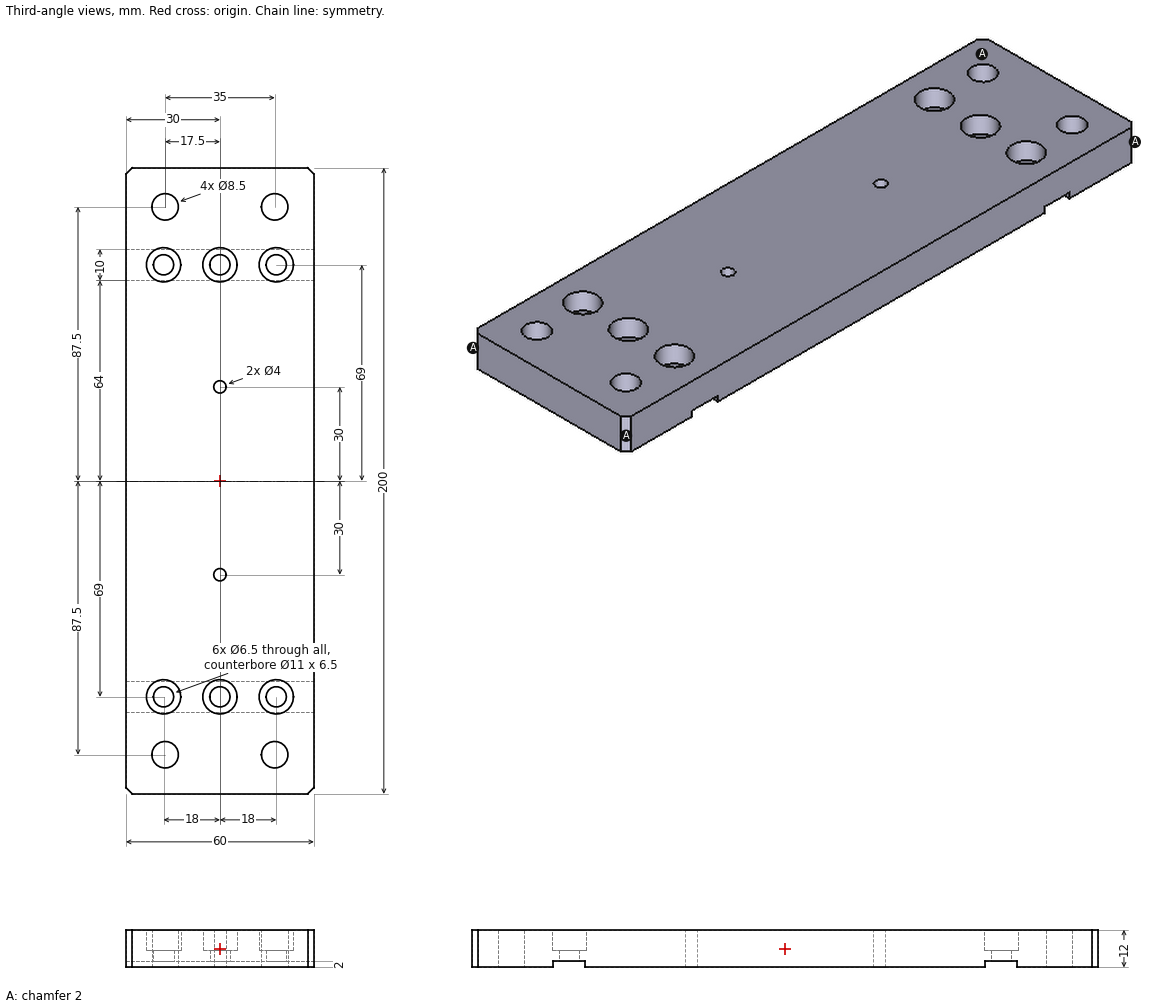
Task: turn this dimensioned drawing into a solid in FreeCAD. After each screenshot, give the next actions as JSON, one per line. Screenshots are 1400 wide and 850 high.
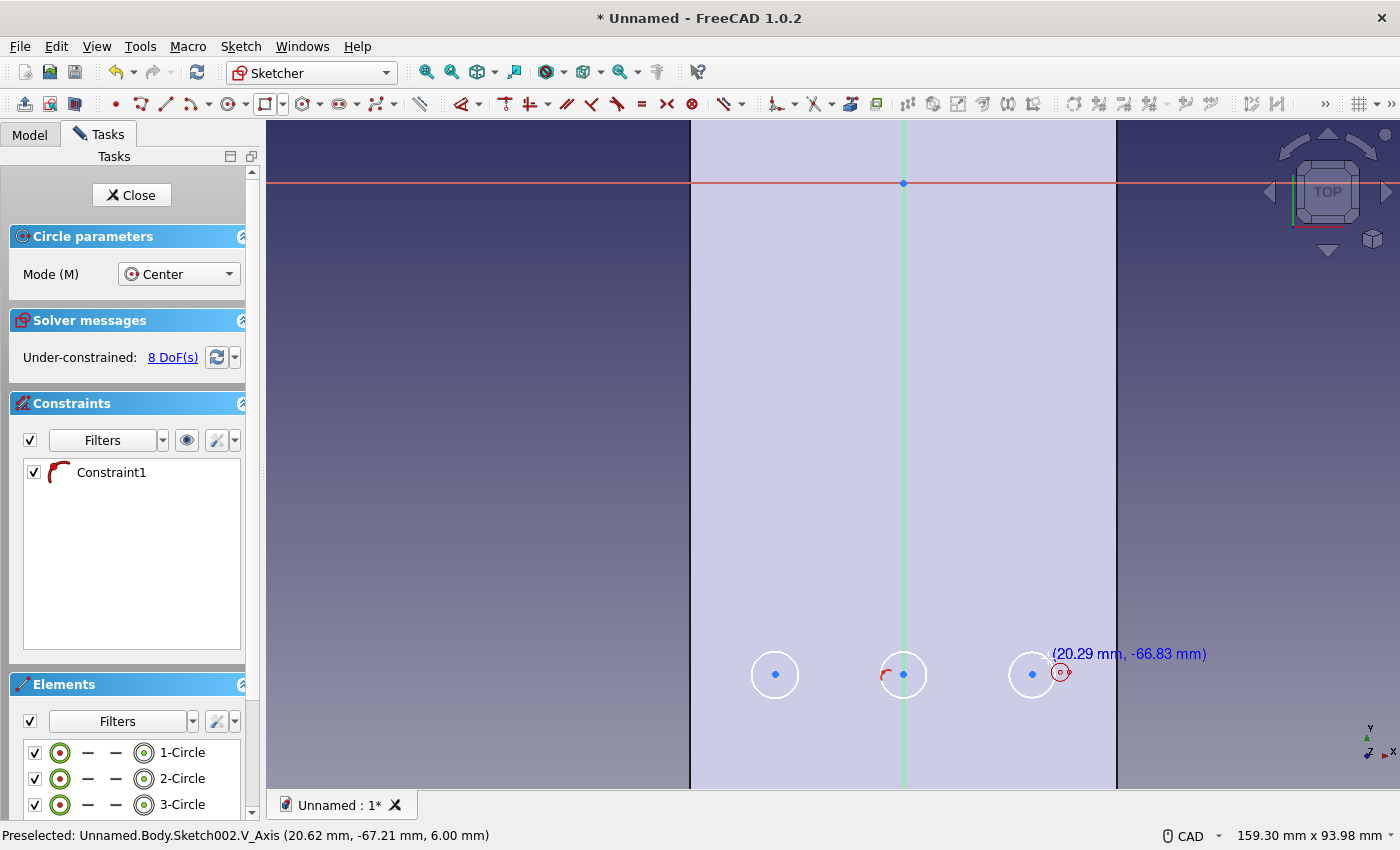
{"action": "scroll", "coordinate": [651, 676], "scroll_direction": "down", "scroll_amount": 4}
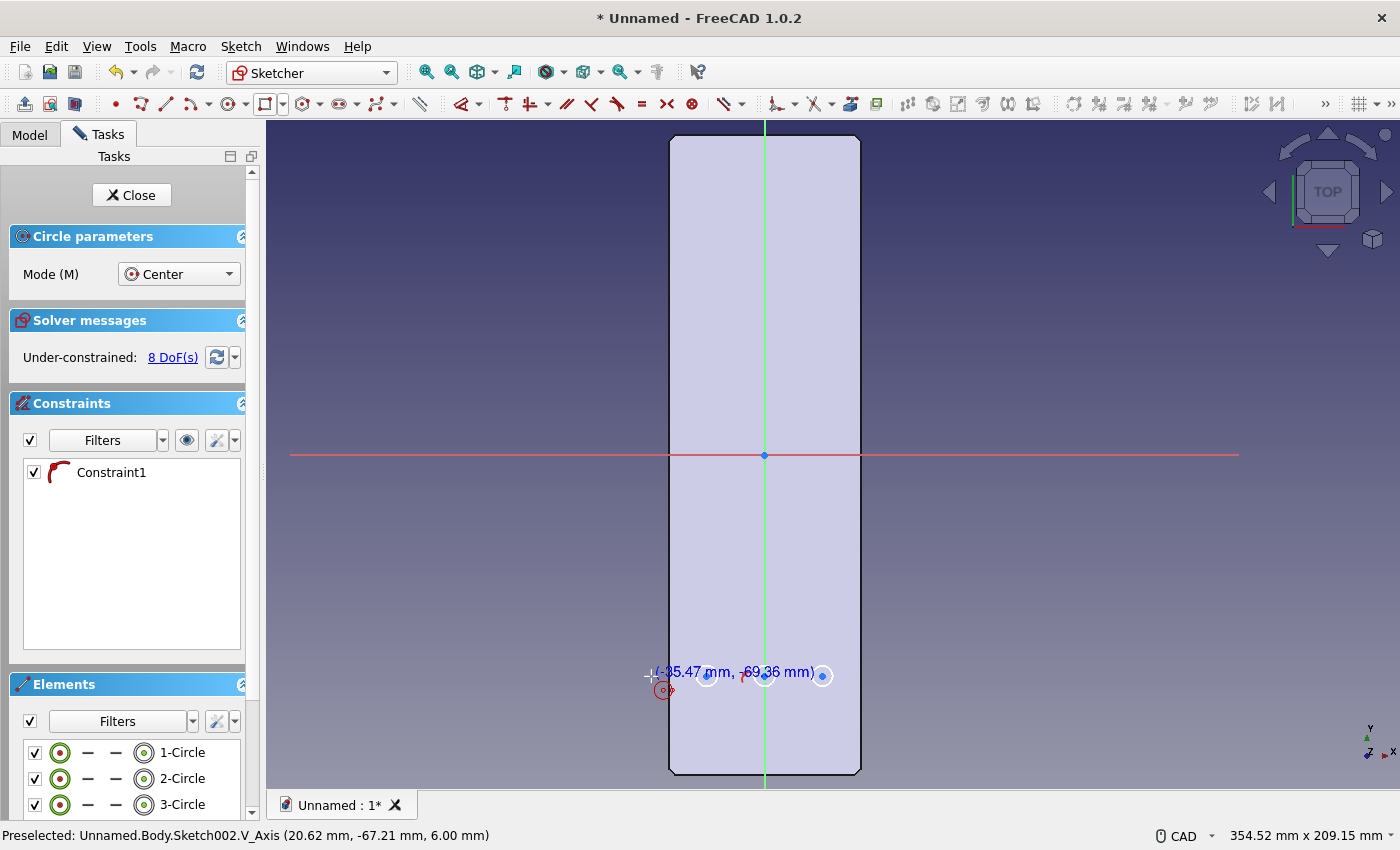
{"action": "scroll", "coordinate": [822, 234], "scroll_direction": "up", "scroll_amount": 4}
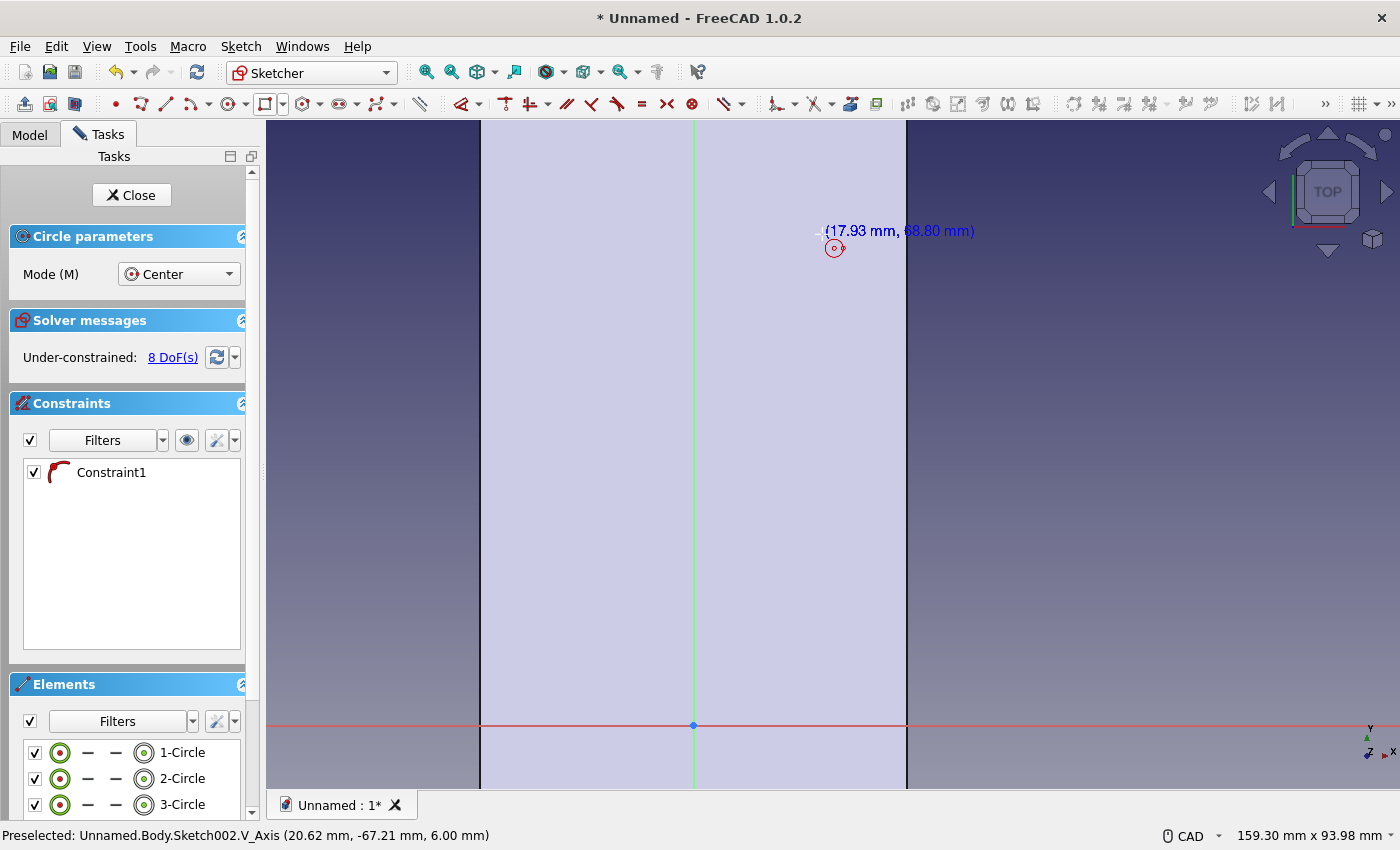
{"action": "left_click", "coordinate": [822, 235]}
{"action": "left_click", "coordinate": [838, 218]}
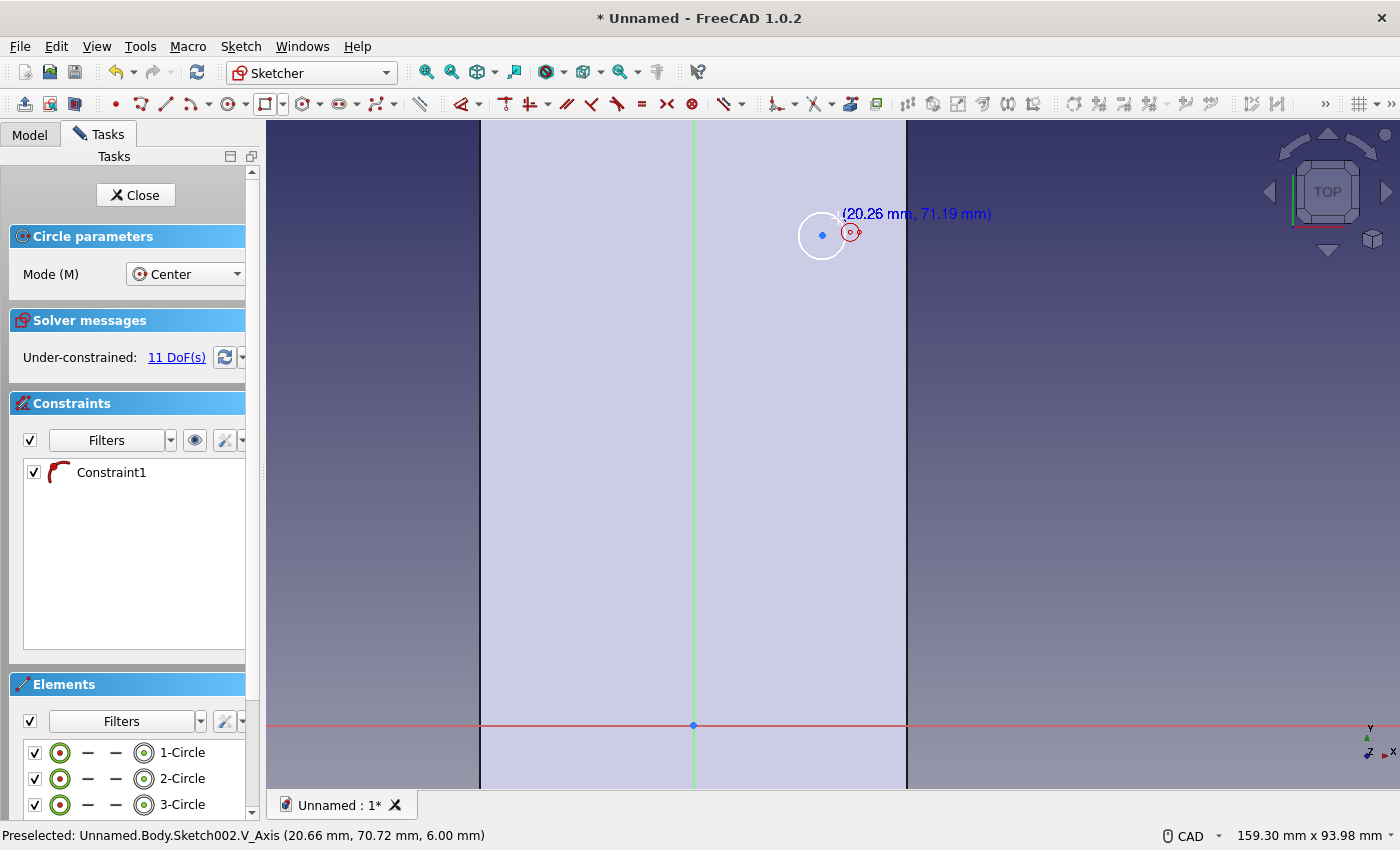
{"action": "left_click", "coordinate": [694, 235]}
{"action": "left_click", "coordinate": [710, 218]}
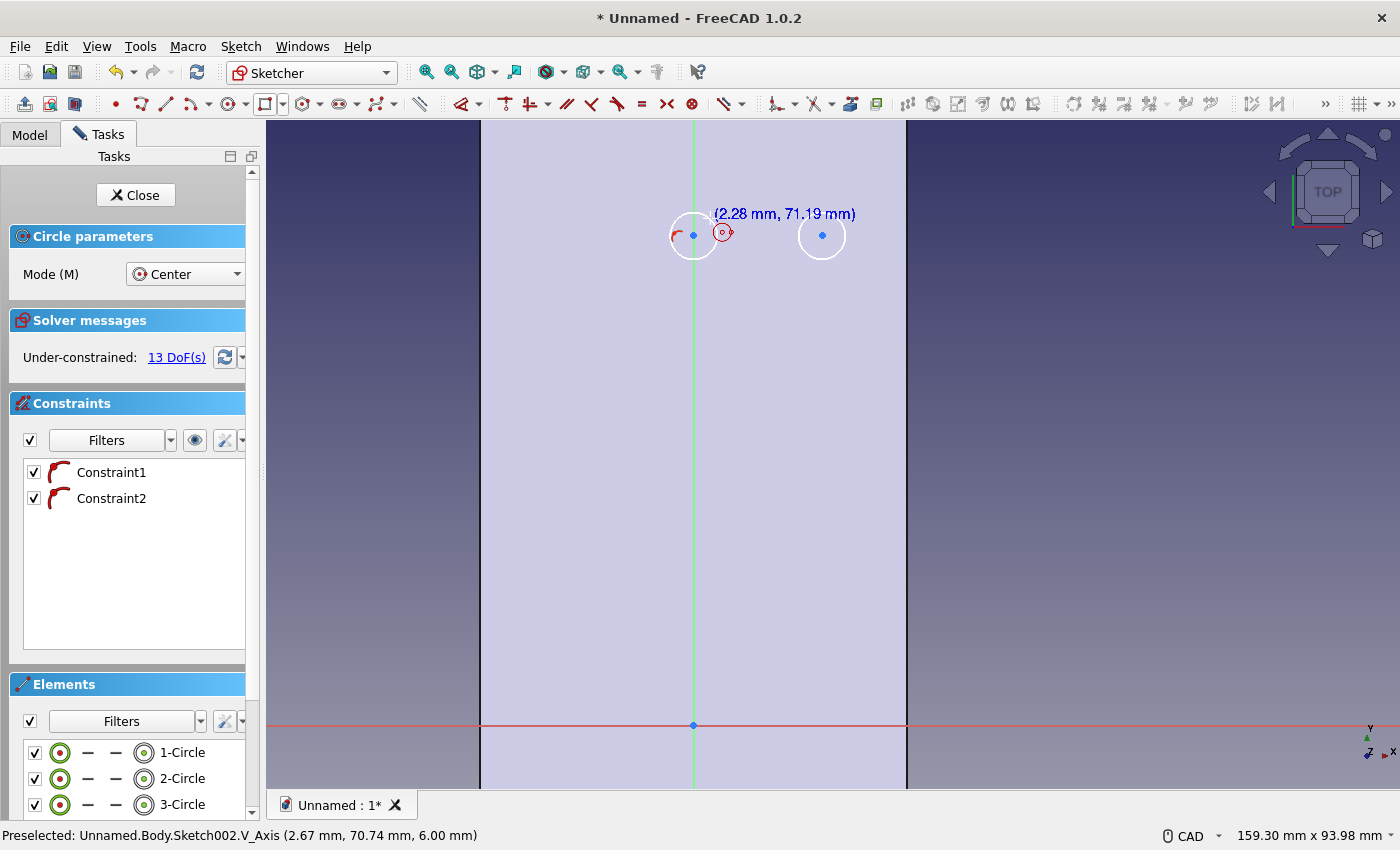
{"action": "left_click", "coordinate": [566, 235]}
{"action": "left_click", "coordinate": [582, 218]}
{"action": "key", "text": "Escape"}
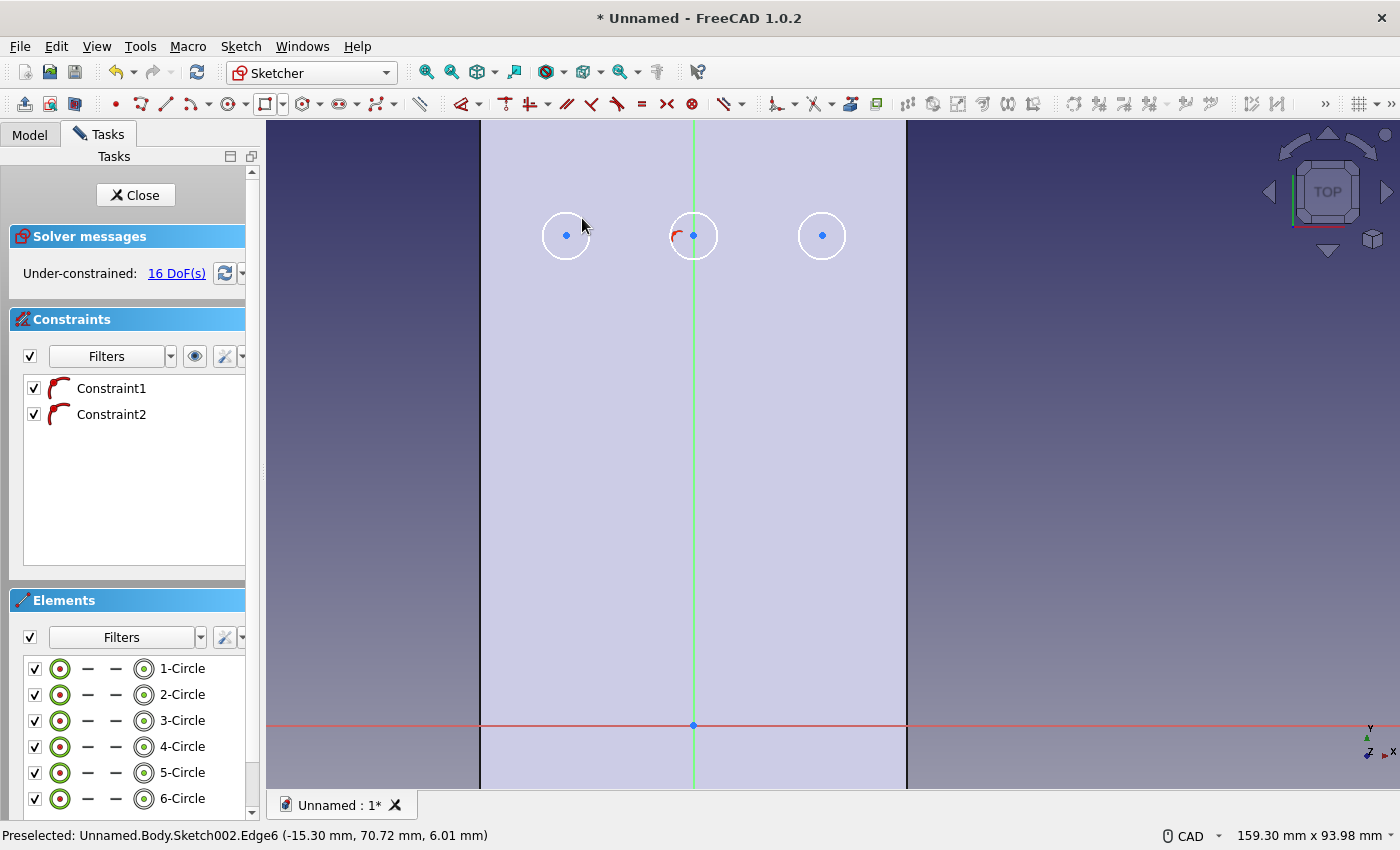
{"action": "scroll", "coordinate": [822, 233], "scroll_direction": "down", "scroll_amount": 4}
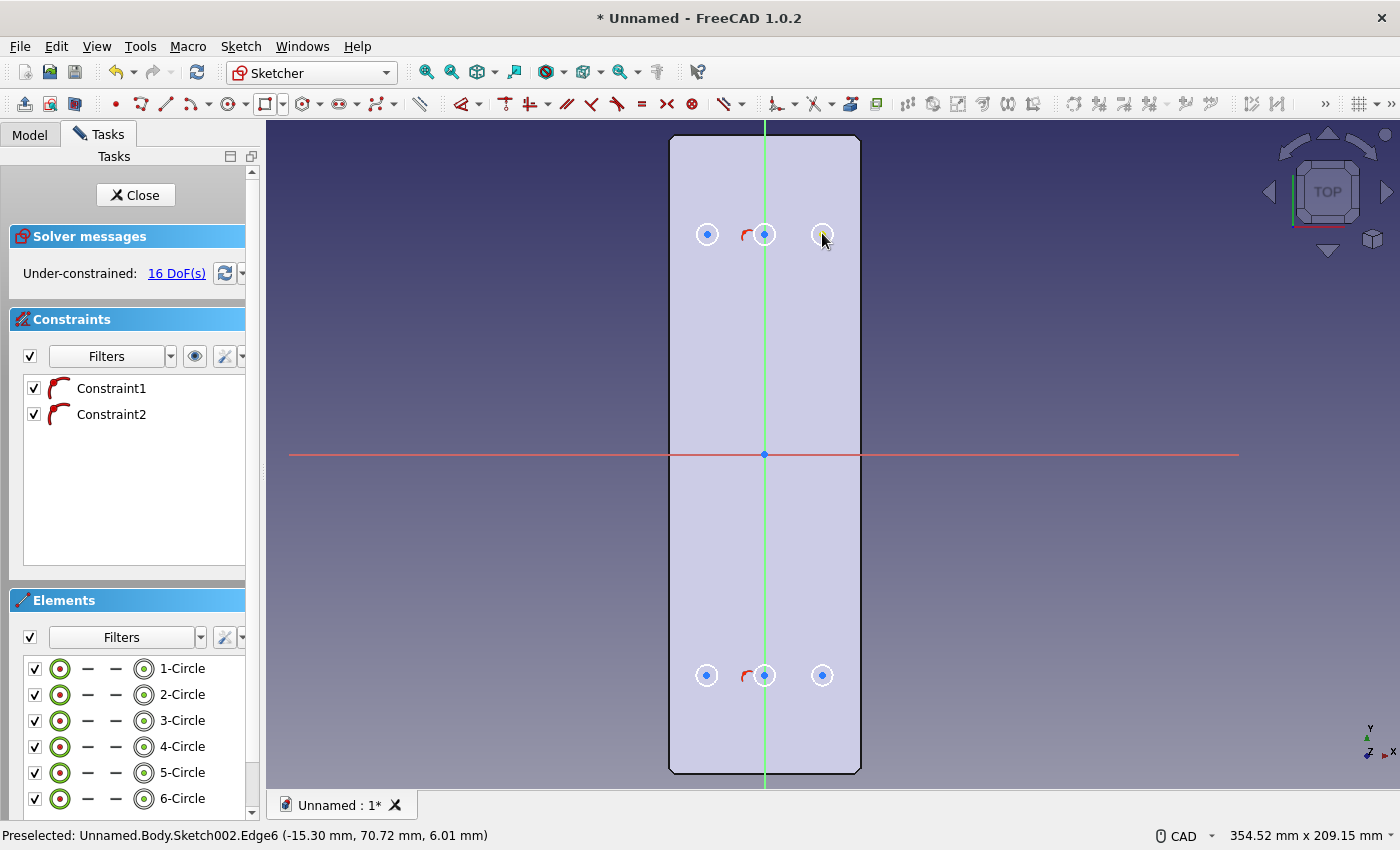
{"action": "scroll", "coordinate": [714, 668], "scroll_direction": "up", "scroll_amount": 2}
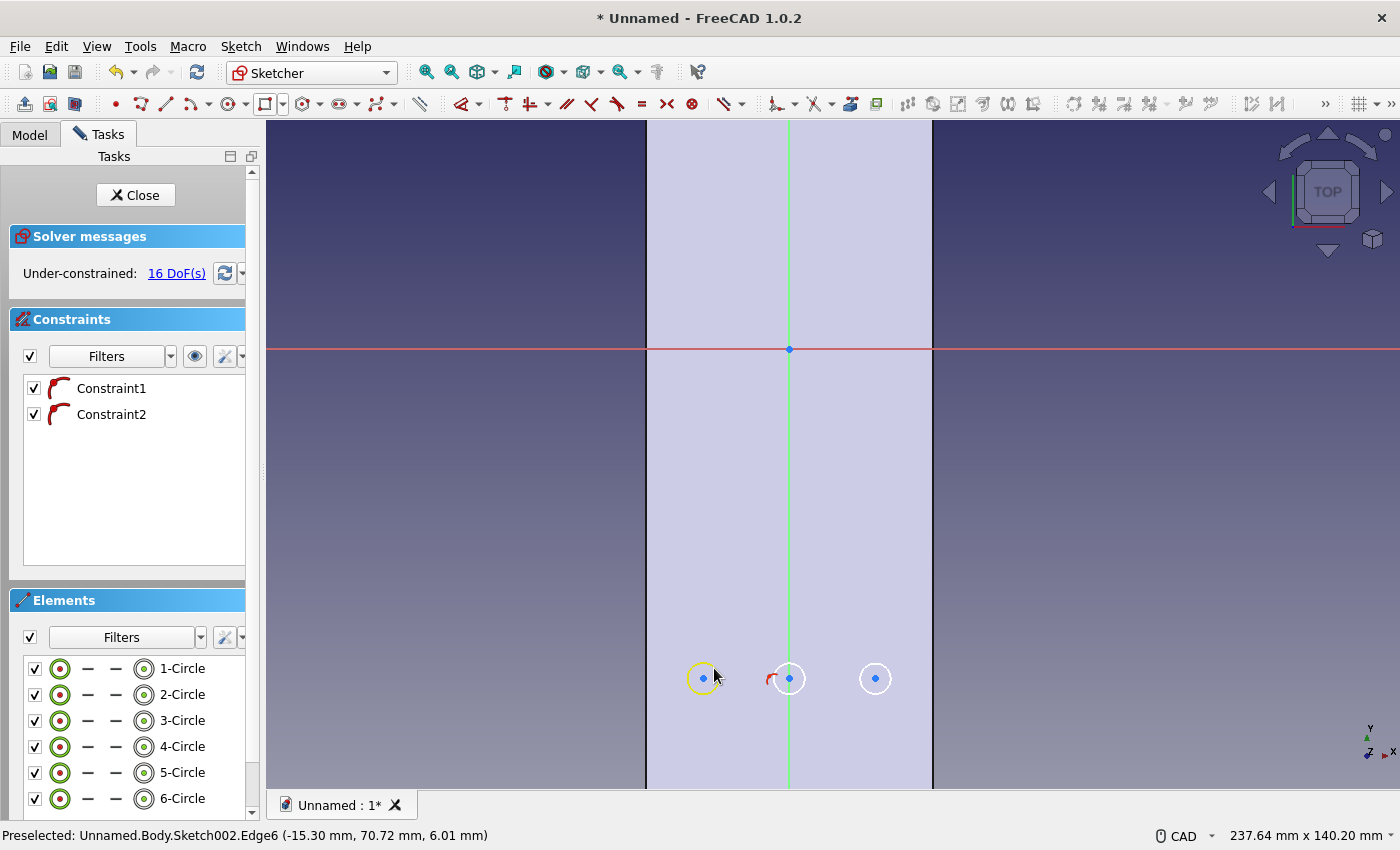
{"action": "left_click", "coordinate": [714, 668]}